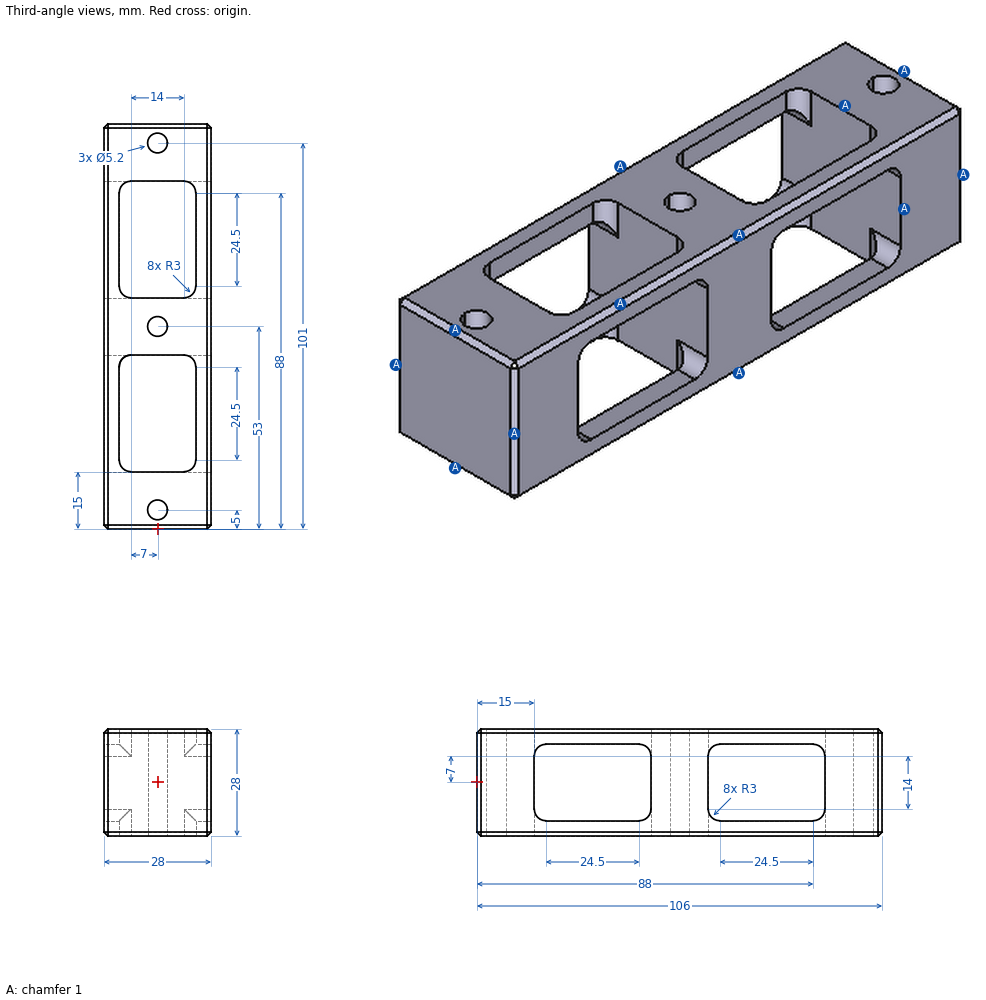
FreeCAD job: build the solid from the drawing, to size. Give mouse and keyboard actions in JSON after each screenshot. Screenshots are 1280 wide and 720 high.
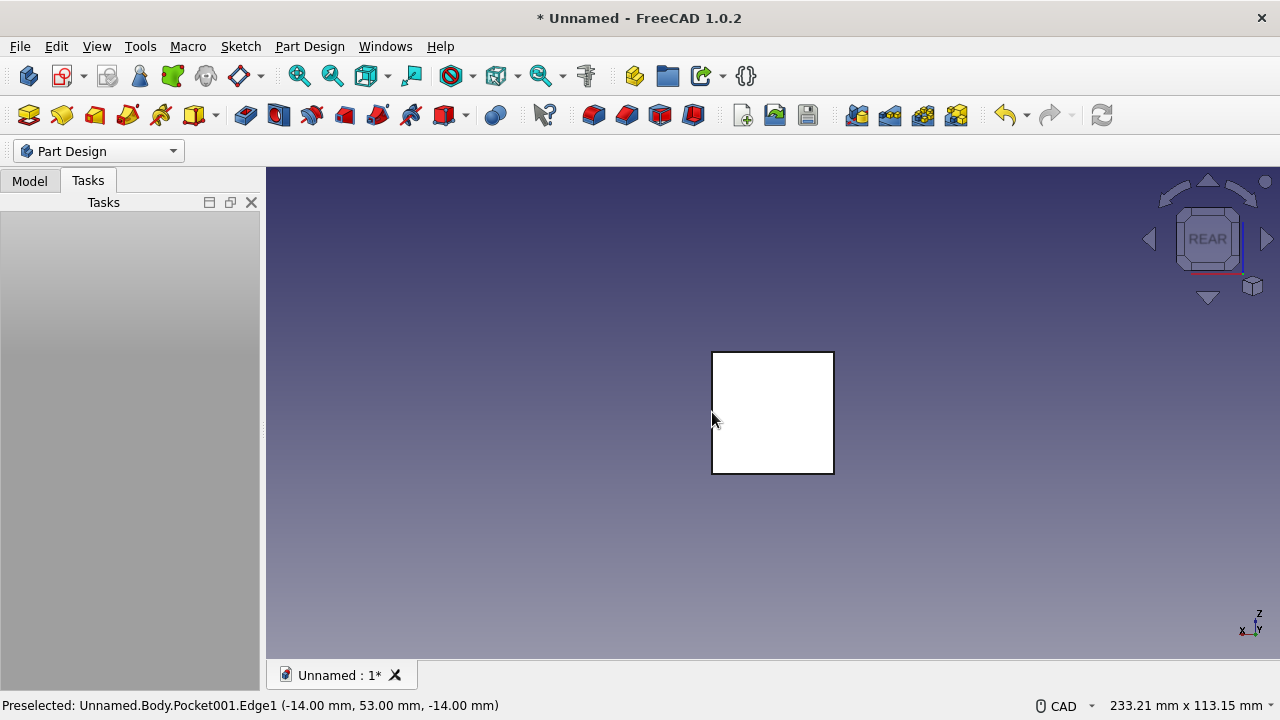
{"action": "left_click", "coordinate": [300, 76]}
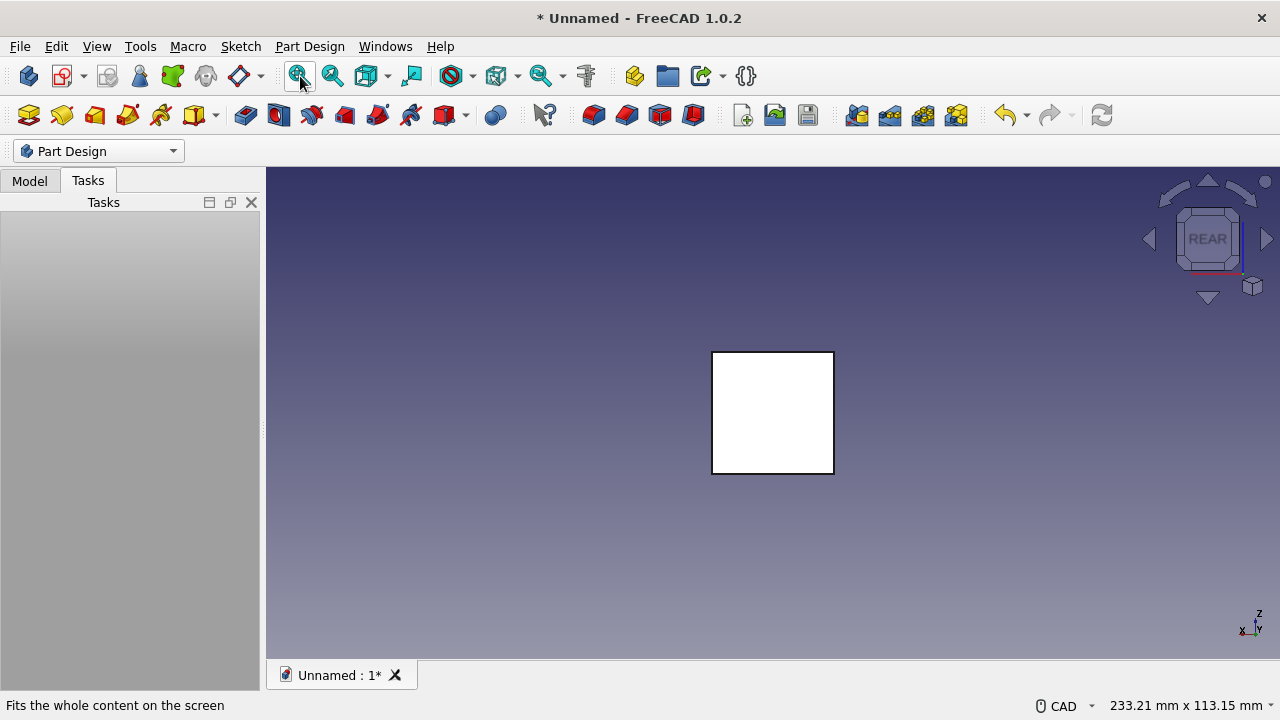
{"action": "left_click", "coordinate": [773, 412], "text": "ctrl"}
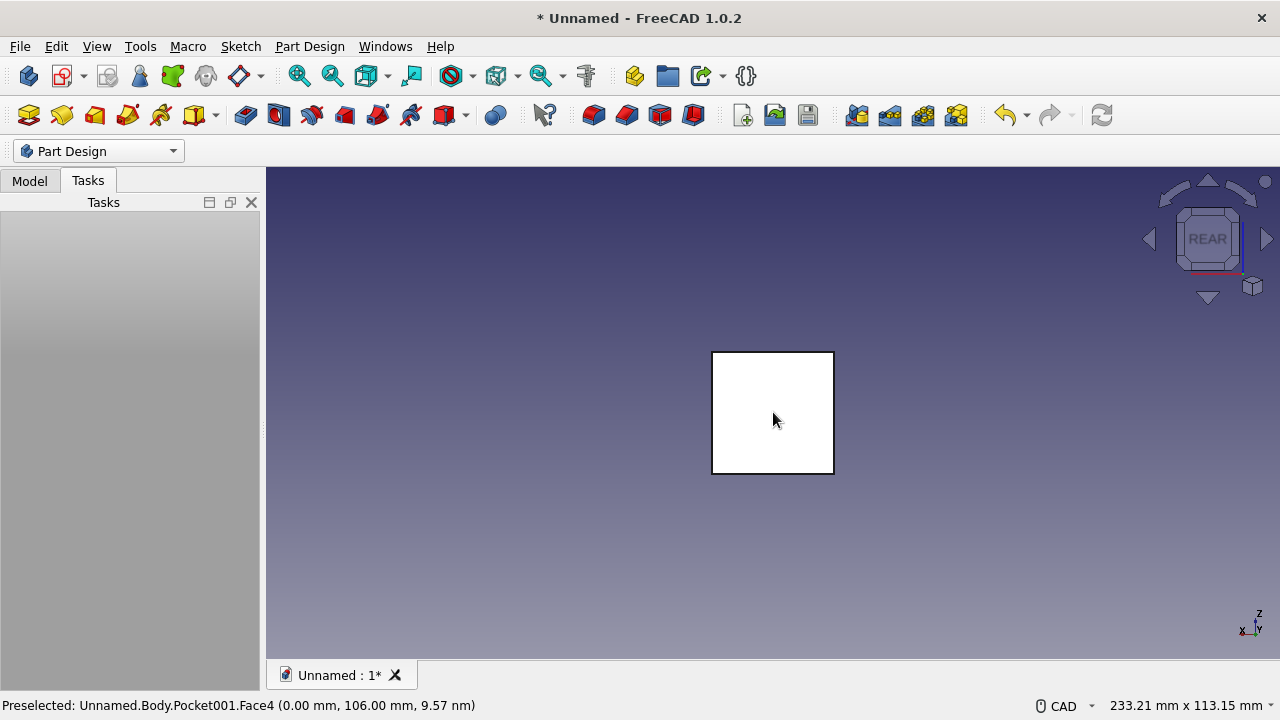
{"action": "left_click", "coordinate": [627, 116]}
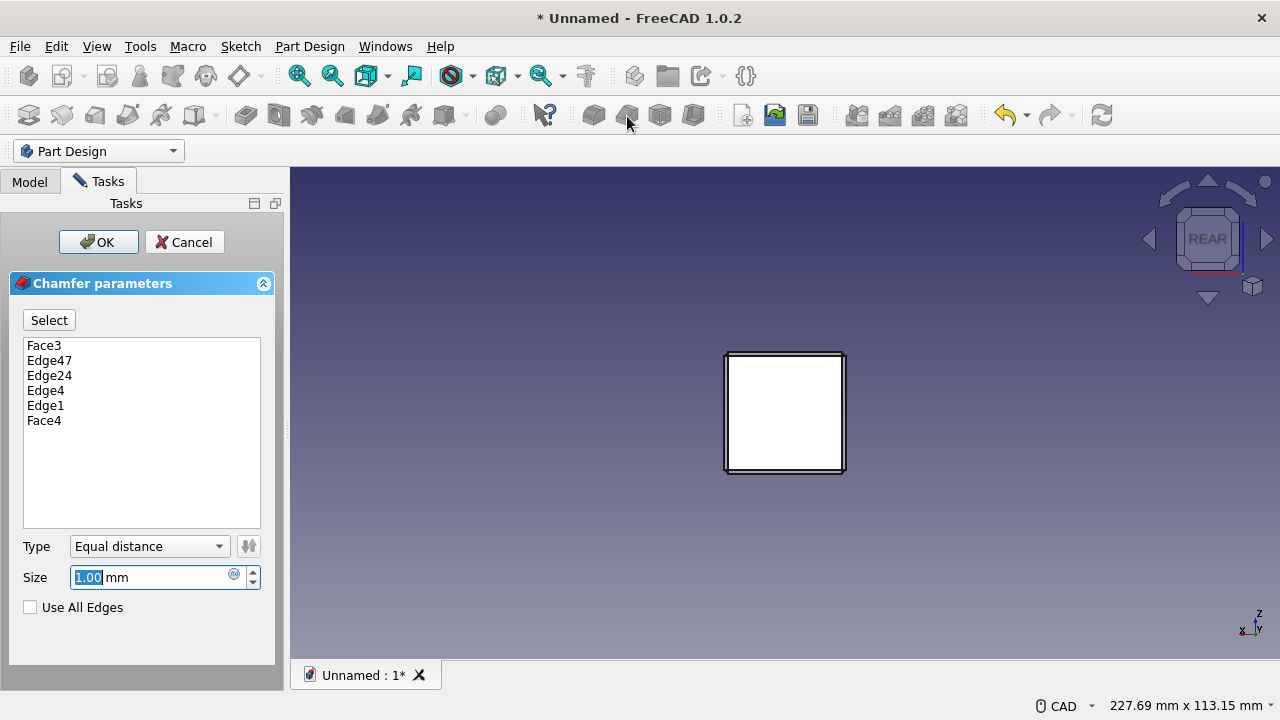
{"action": "type", "text": "1"}
{"action": "key", "text": "Tab"}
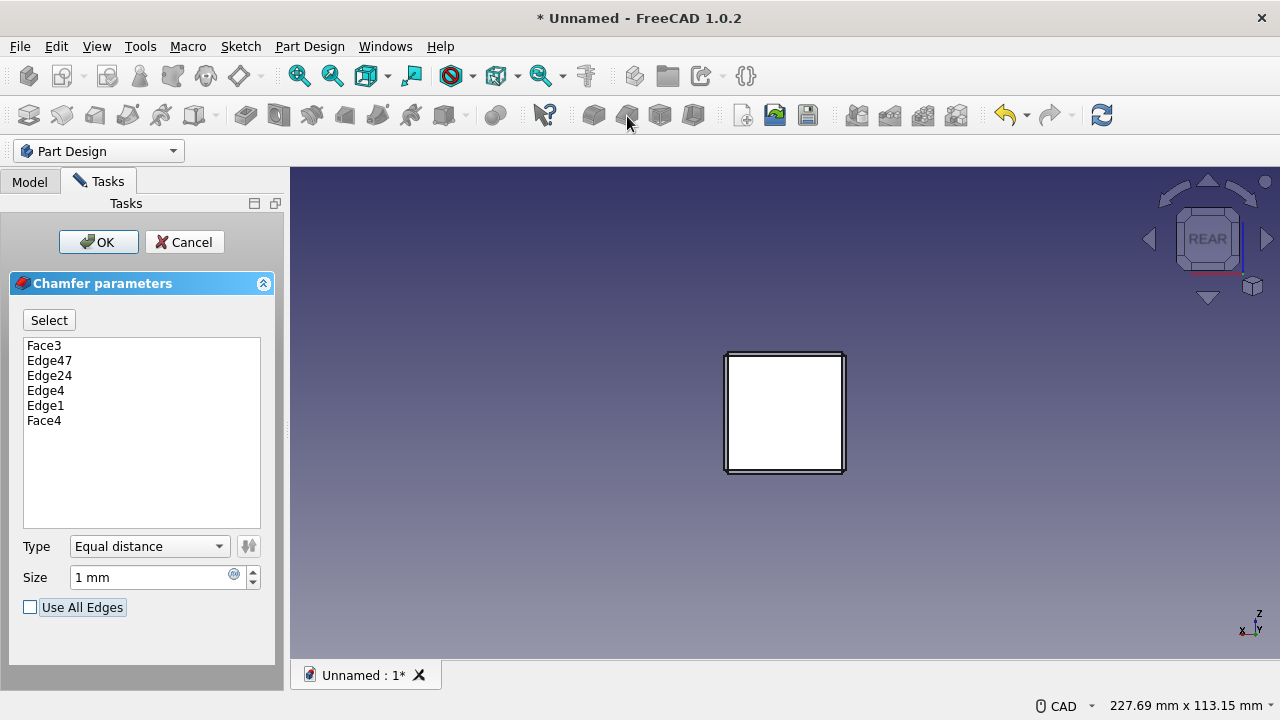
{"action": "left_click", "coordinate": [99, 242]}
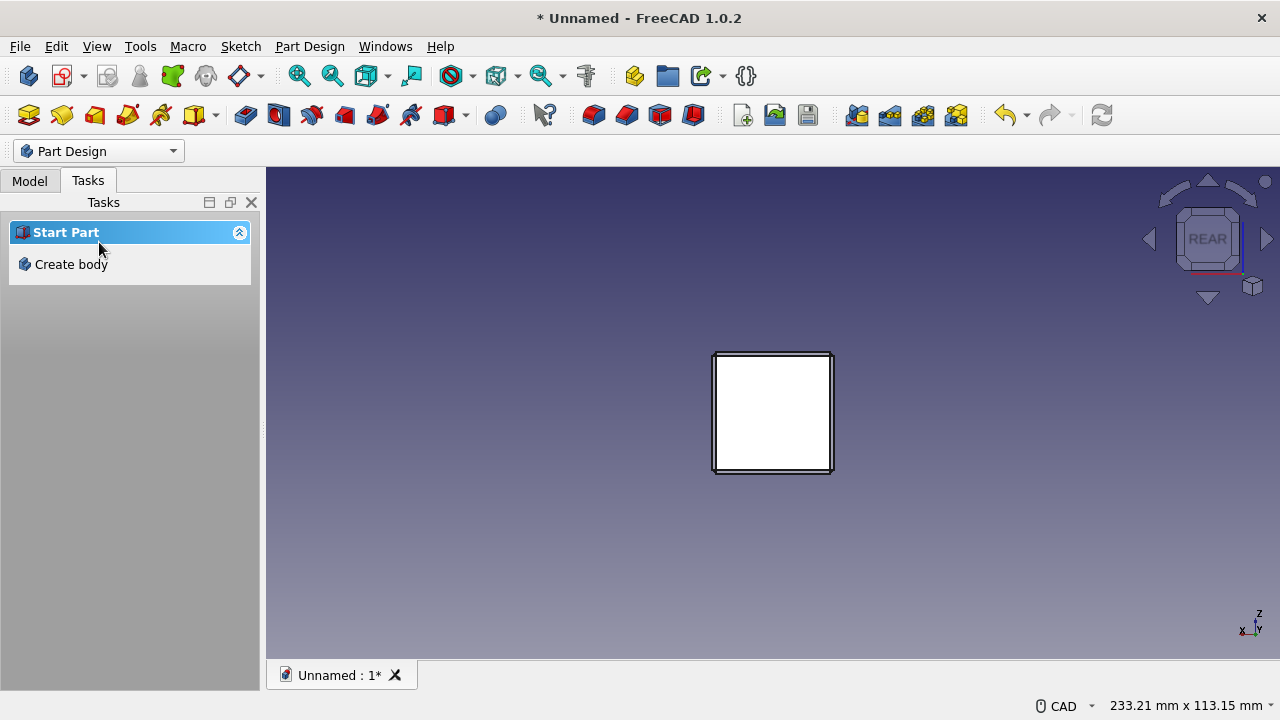
{"action": "key", "text": "0"}